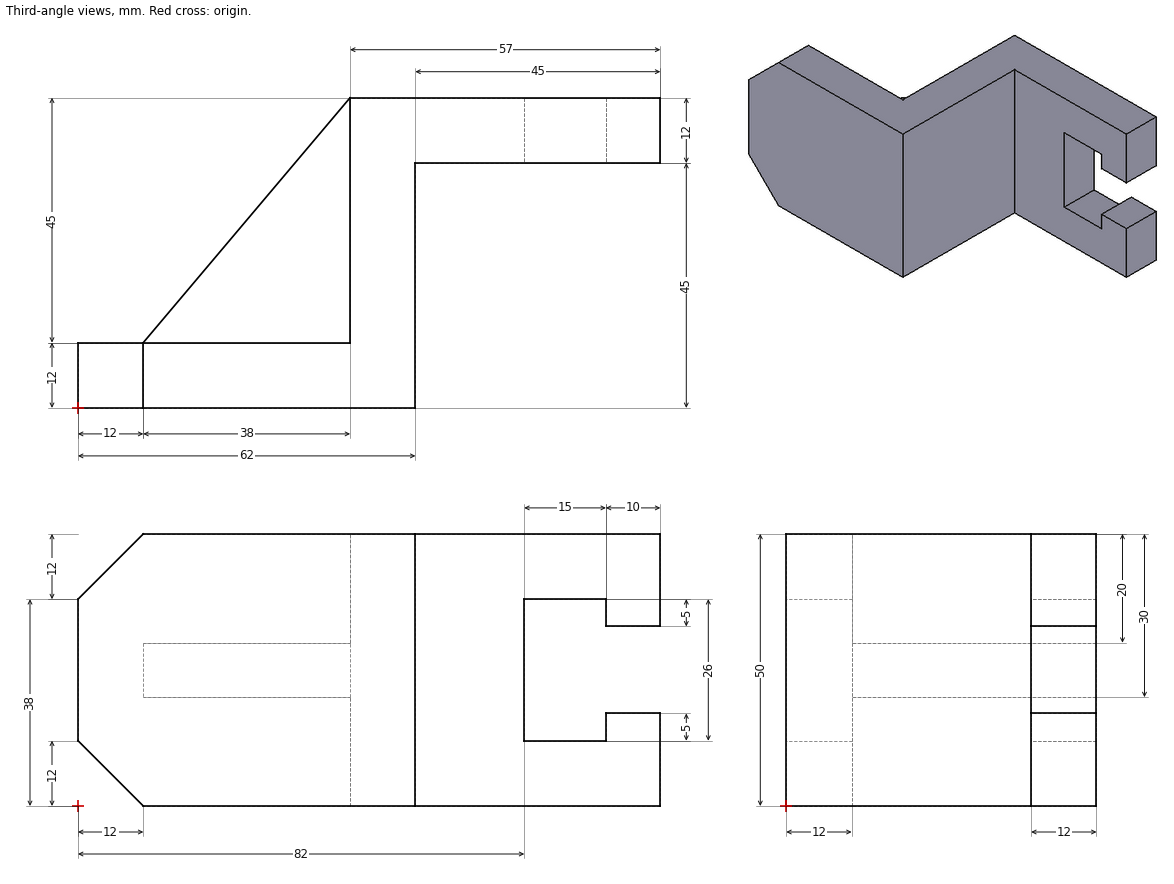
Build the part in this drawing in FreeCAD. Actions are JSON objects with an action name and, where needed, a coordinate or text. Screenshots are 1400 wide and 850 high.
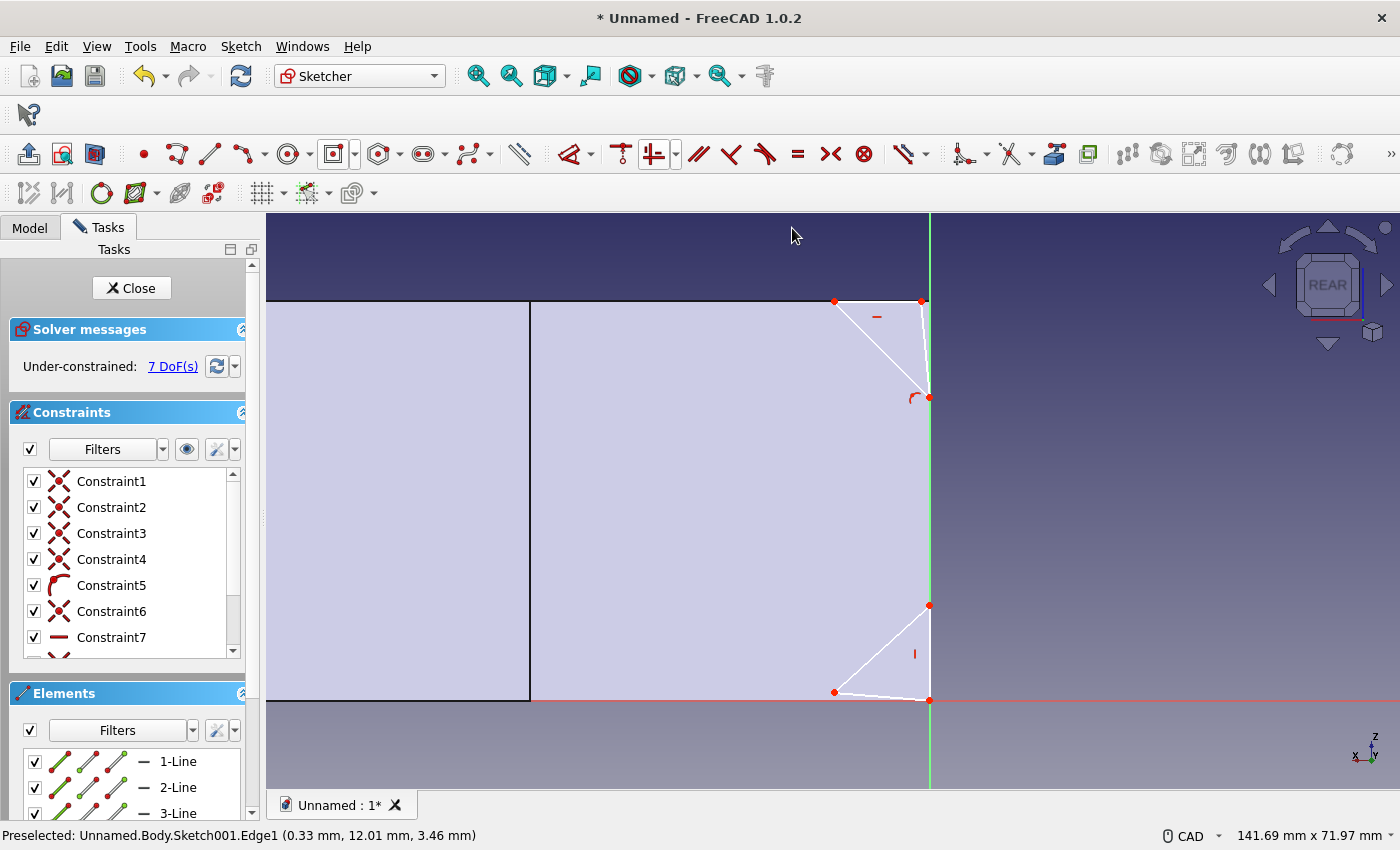
{"action": "left_click", "coordinate": [901, 698]}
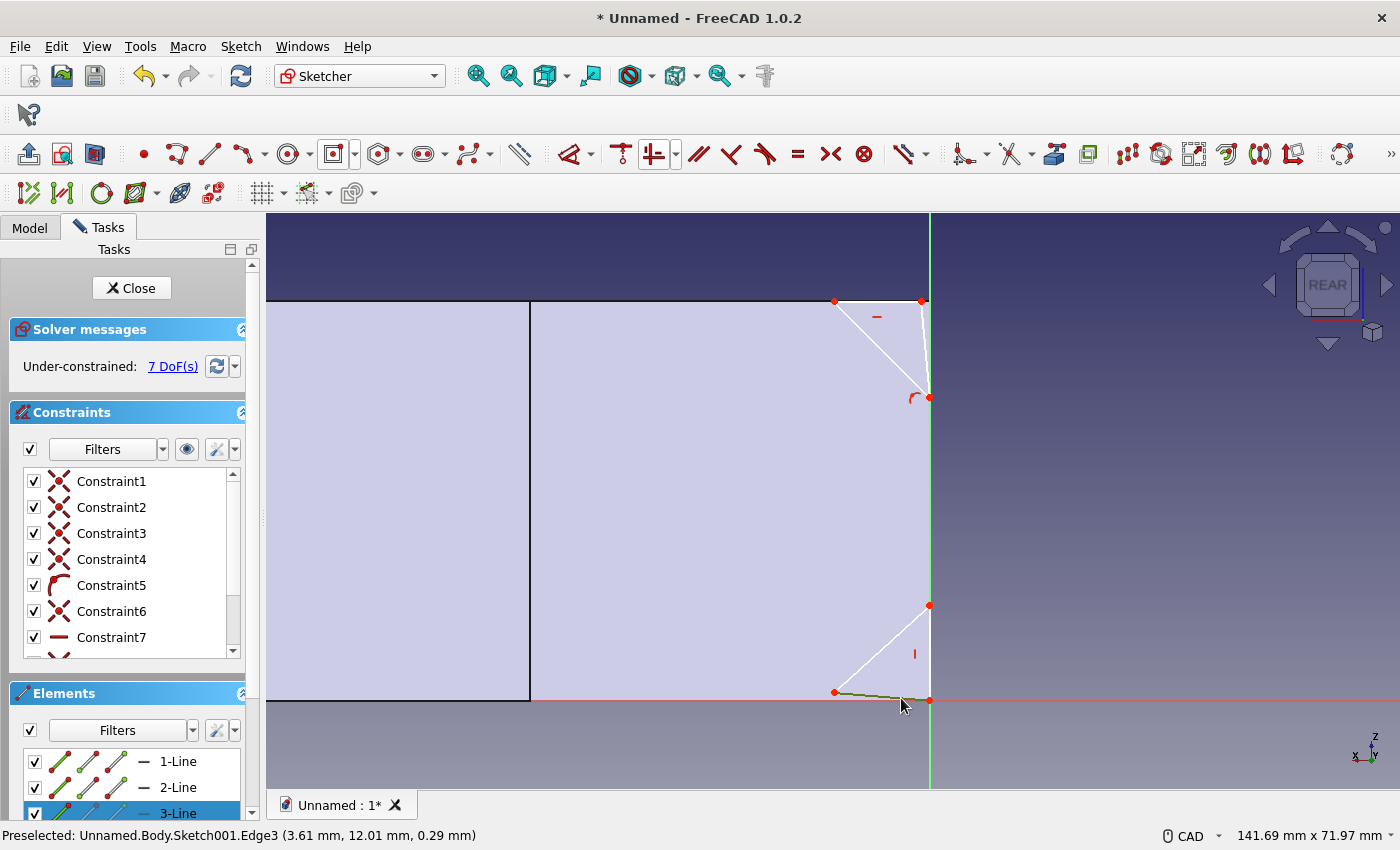
{"action": "key", "text": "h"}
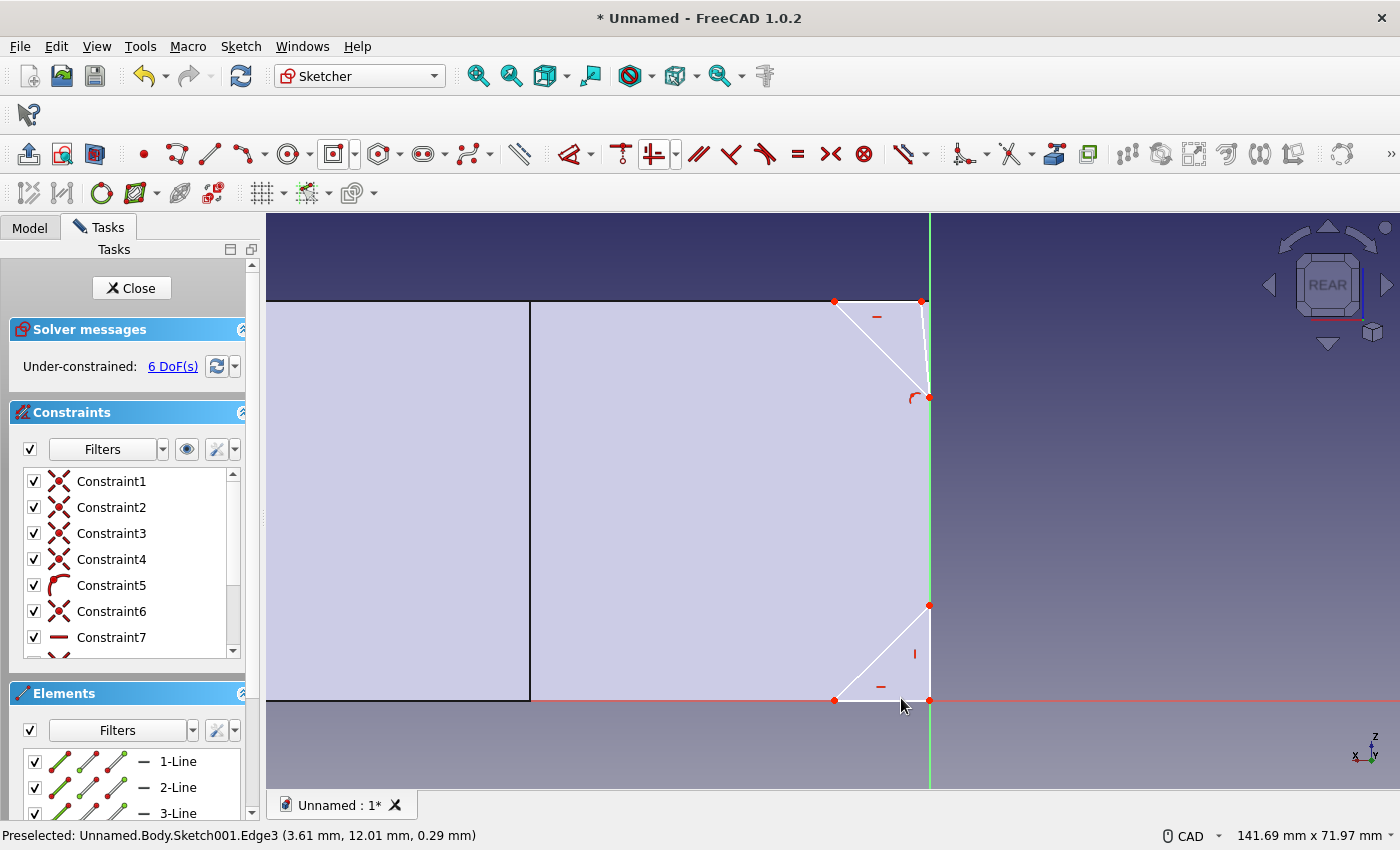
{"action": "left_click", "coordinate": [927, 369]}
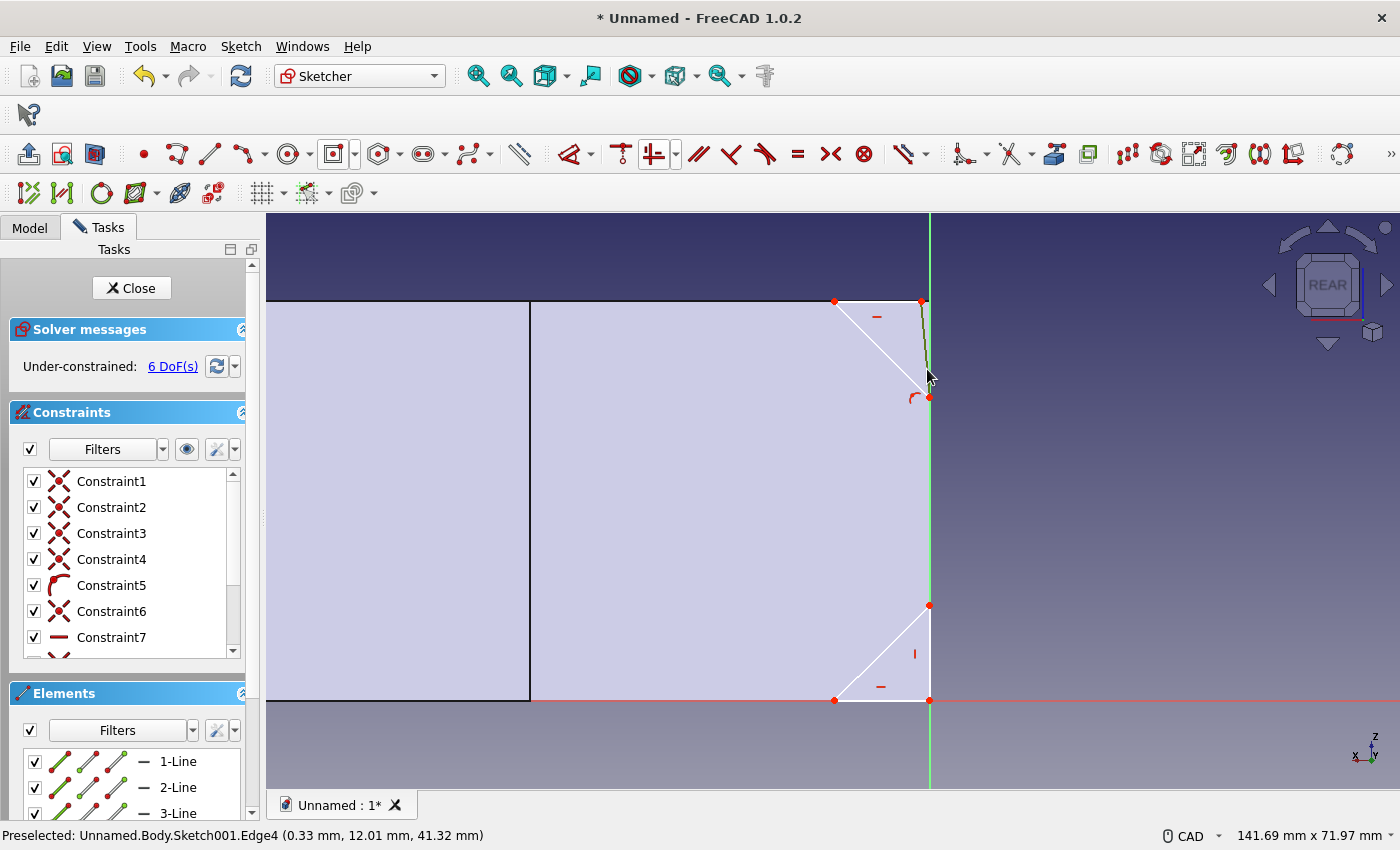
{"action": "key", "text": "v"}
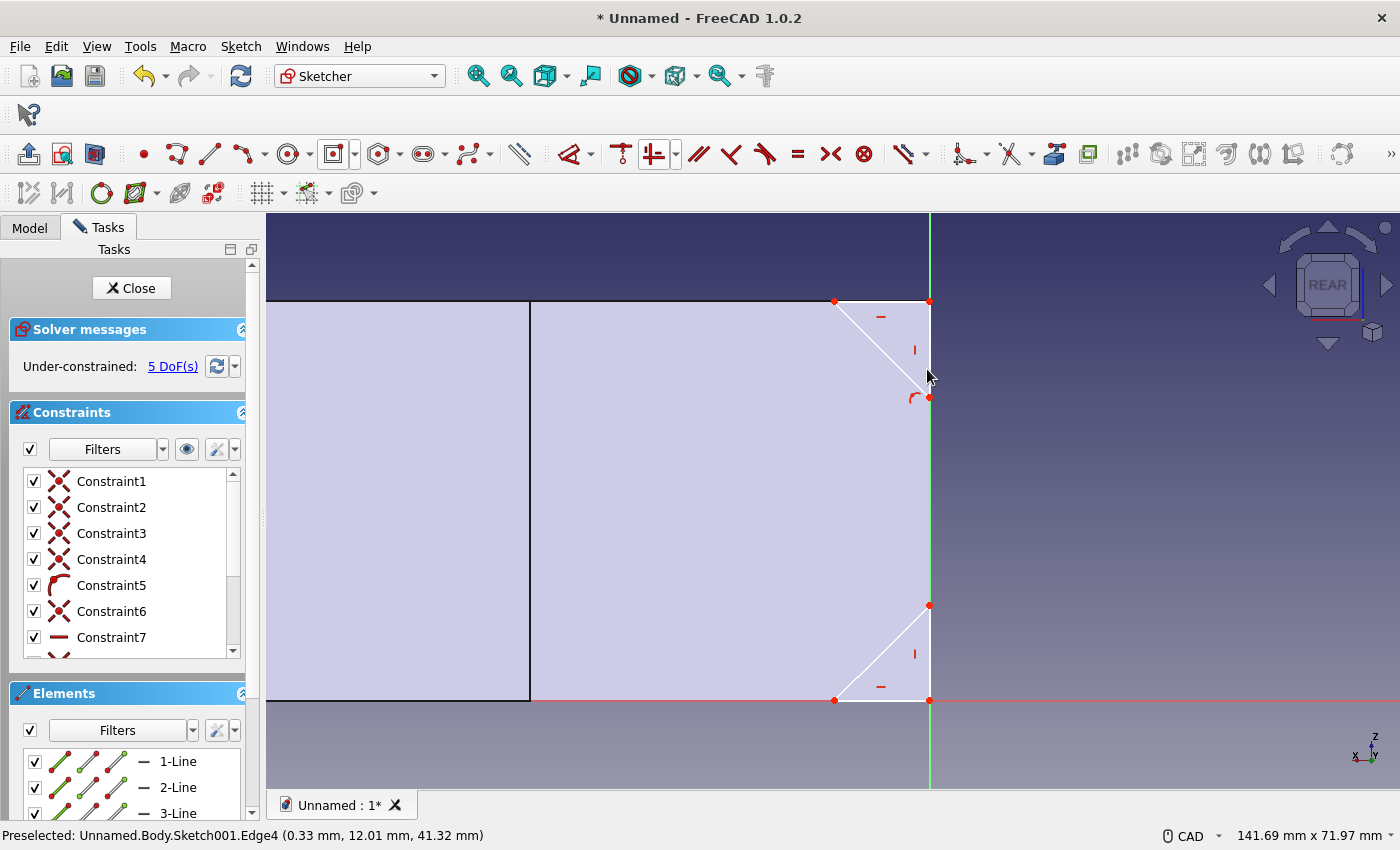
{"action": "left_click", "coordinate": [568, 154]}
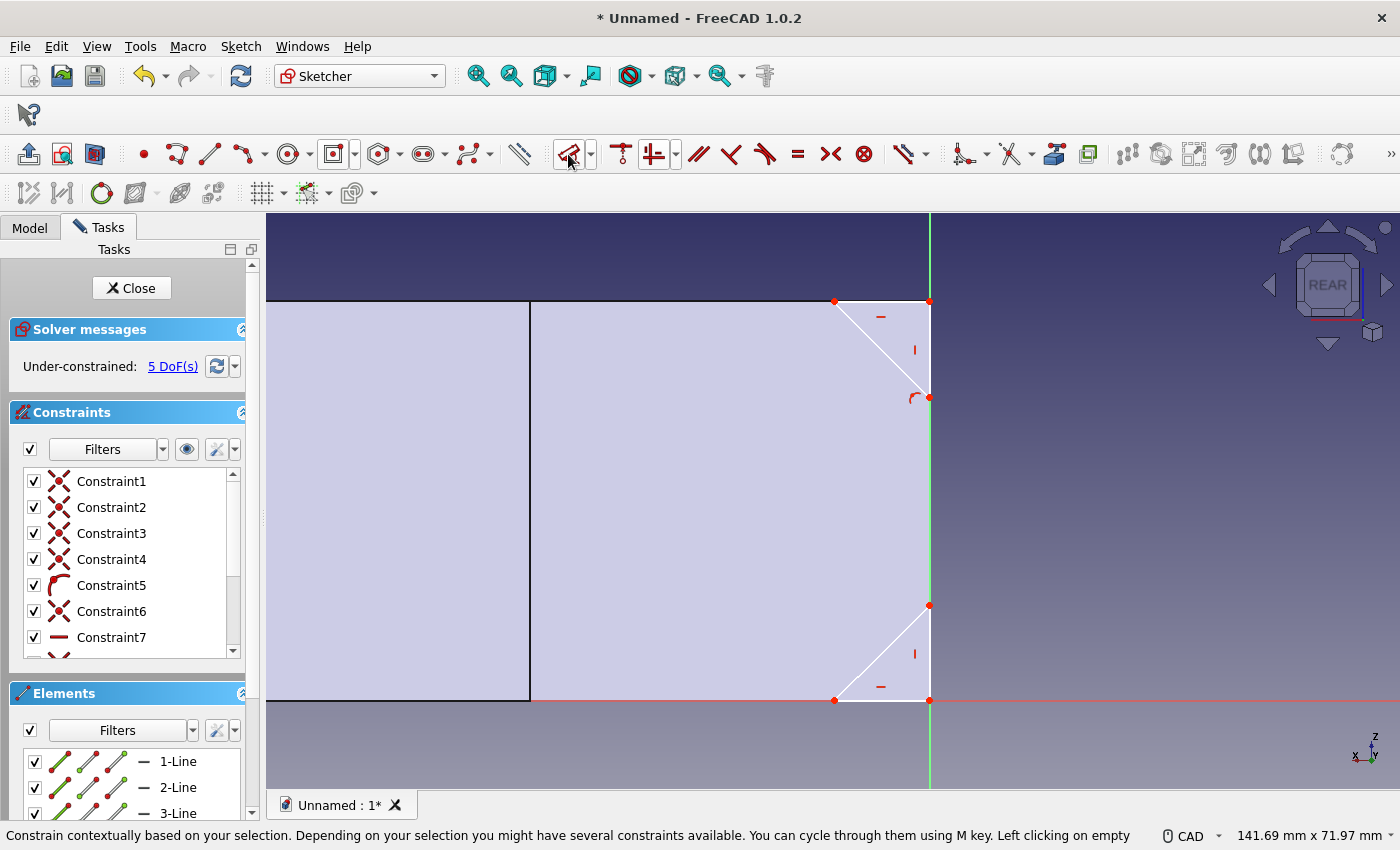
{"action": "left_click", "coordinate": [930, 672]}
{"action": "left_click", "coordinate": [964, 653]}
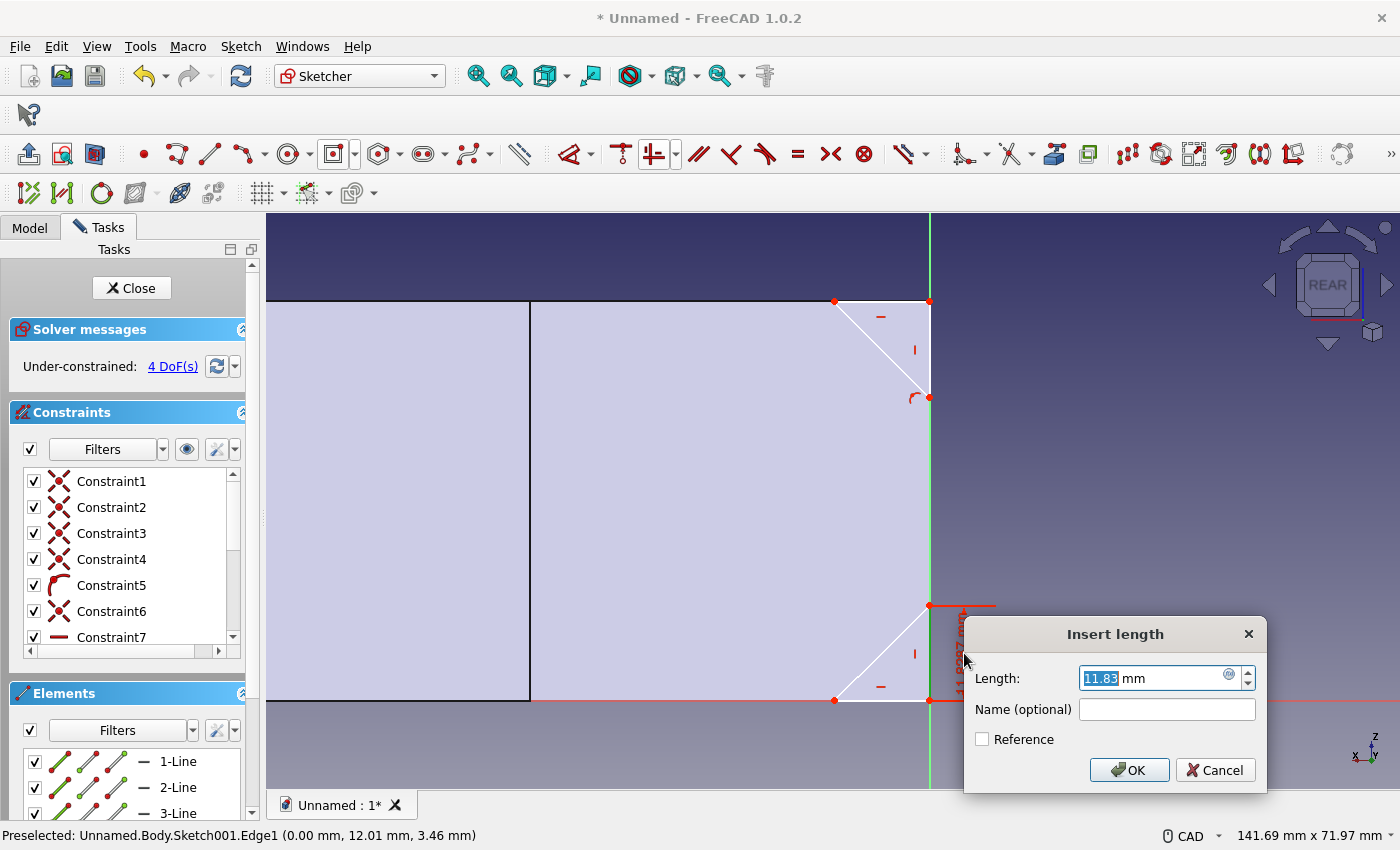
{"action": "type", "text": "12"}
{"action": "key", "text": "Return"}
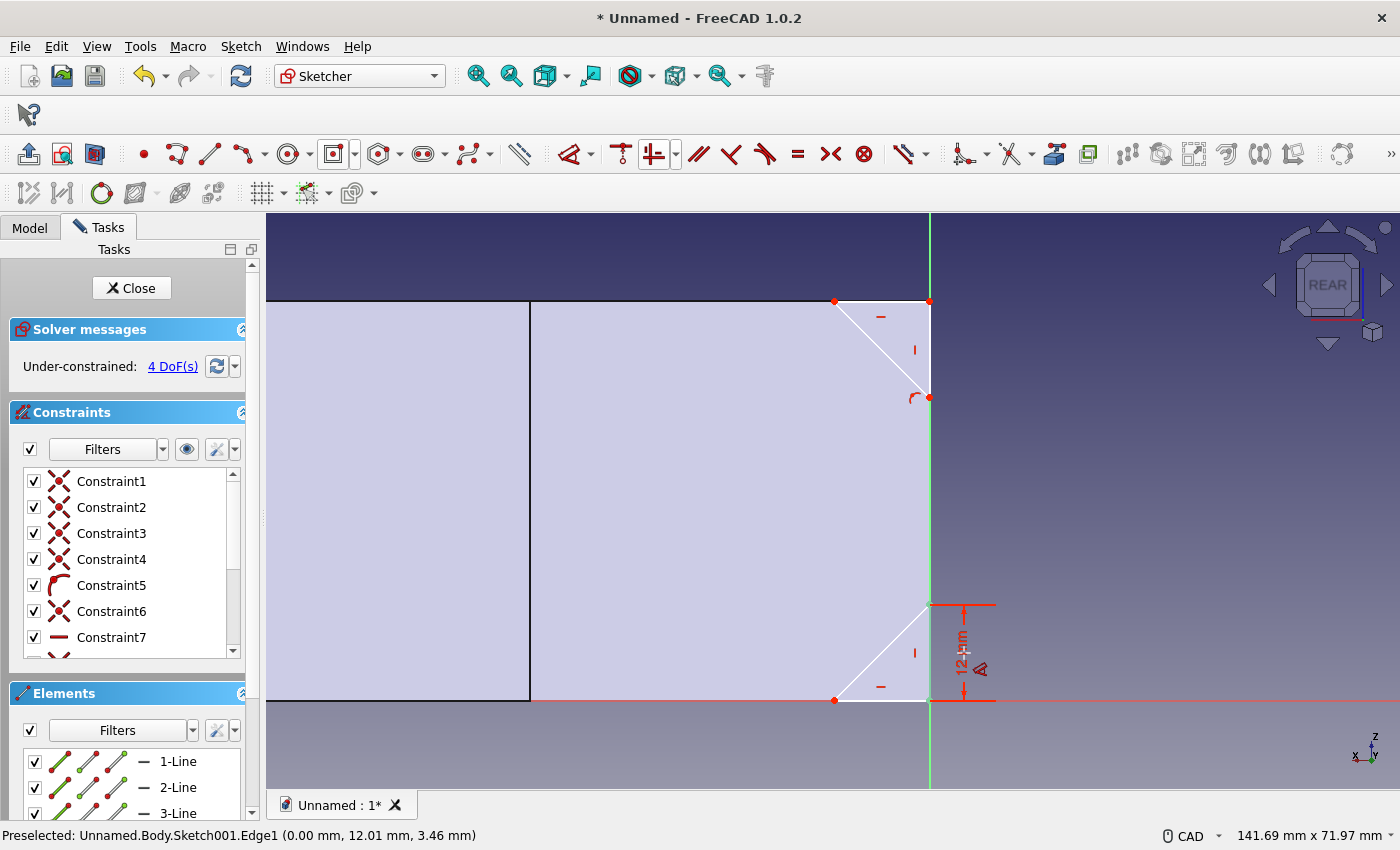
{"action": "left_click", "coordinate": [863, 701]}
{"action": "left_click", "coordinate": [882, 735]}